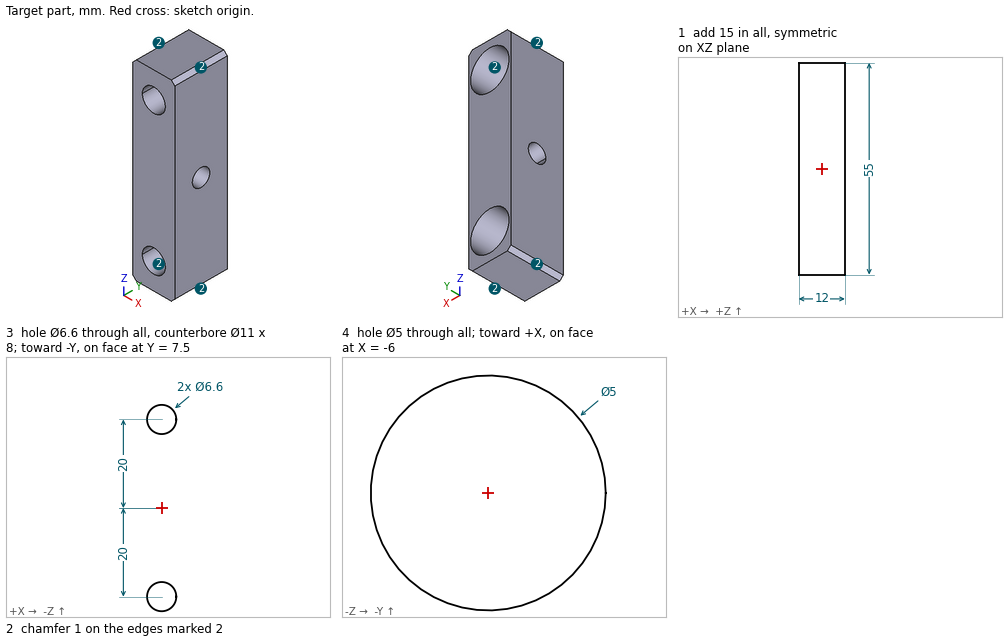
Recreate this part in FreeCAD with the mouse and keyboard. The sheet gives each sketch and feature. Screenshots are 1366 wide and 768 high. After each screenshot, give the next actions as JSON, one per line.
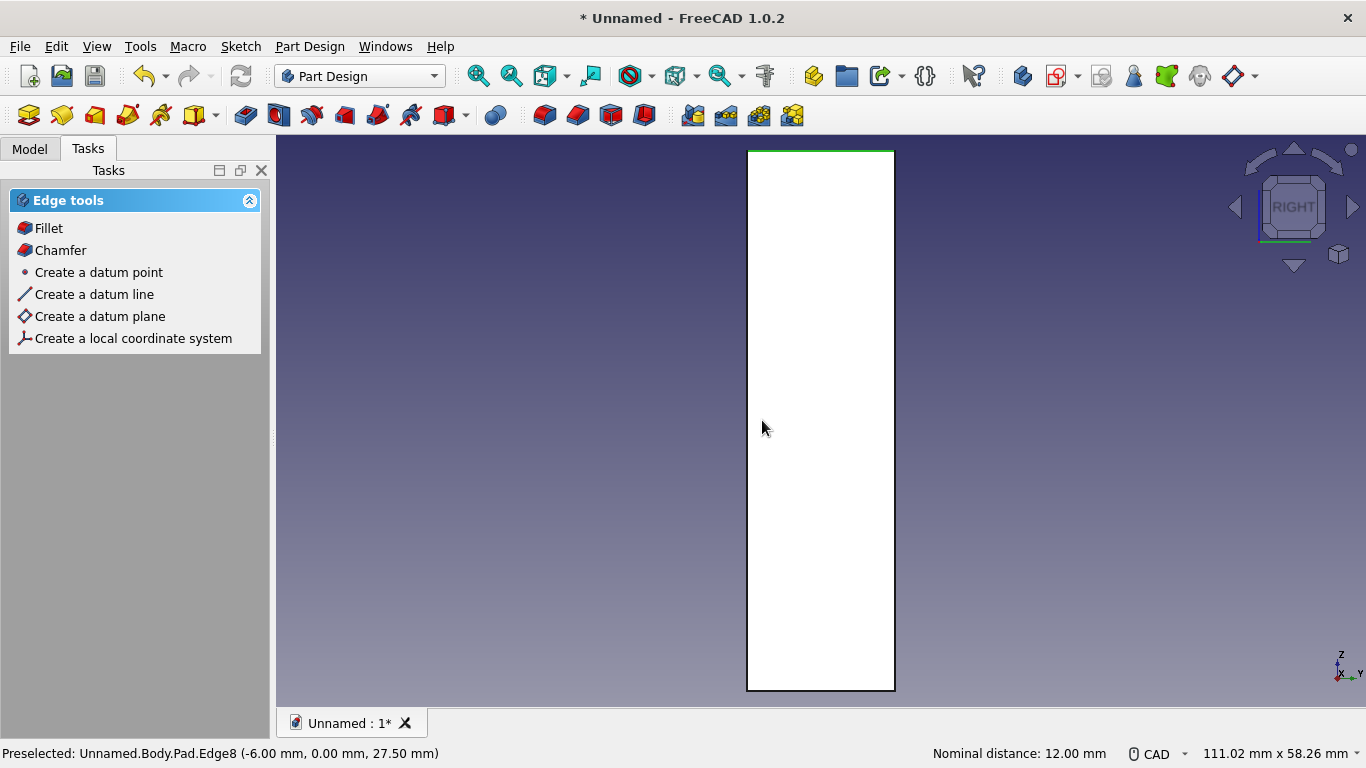
{"action": "key", "text": "5"}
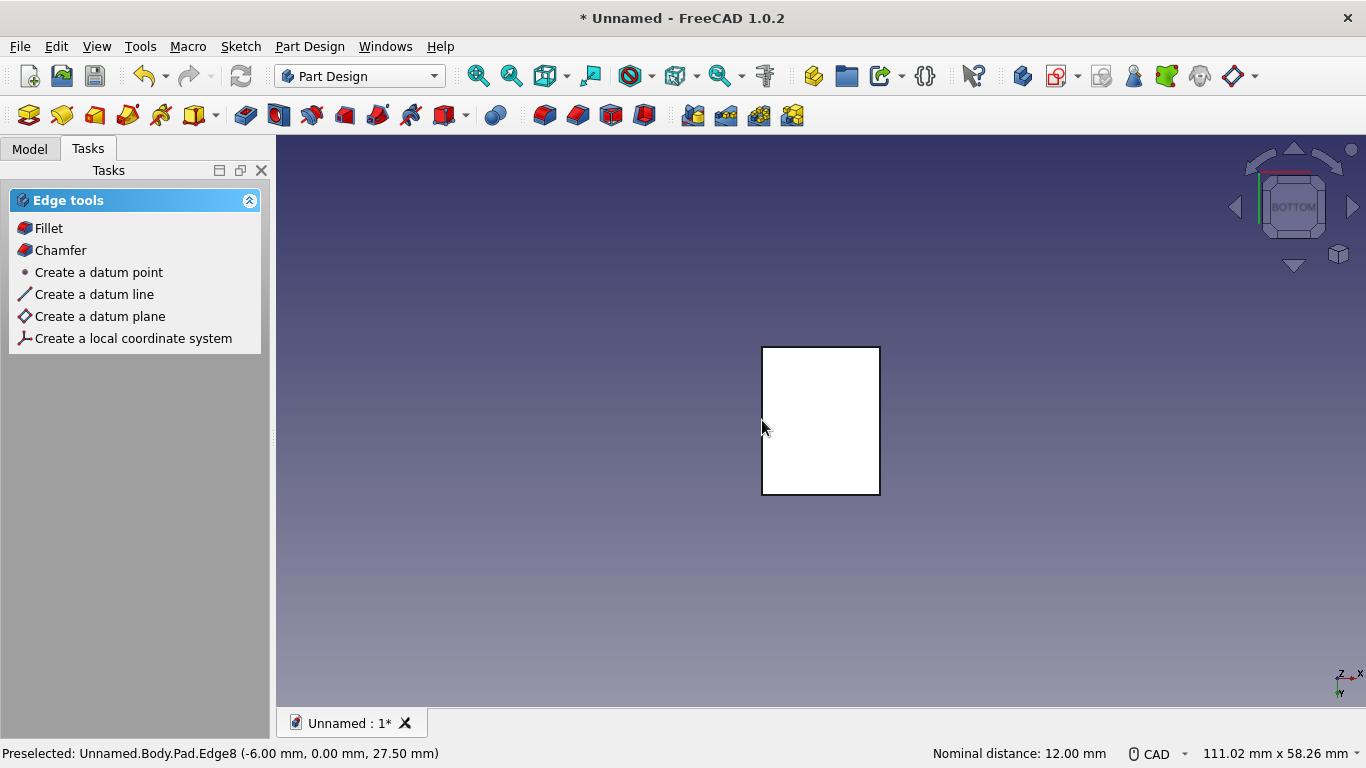
{"action": "left_click", "coordinate": [479, 76]}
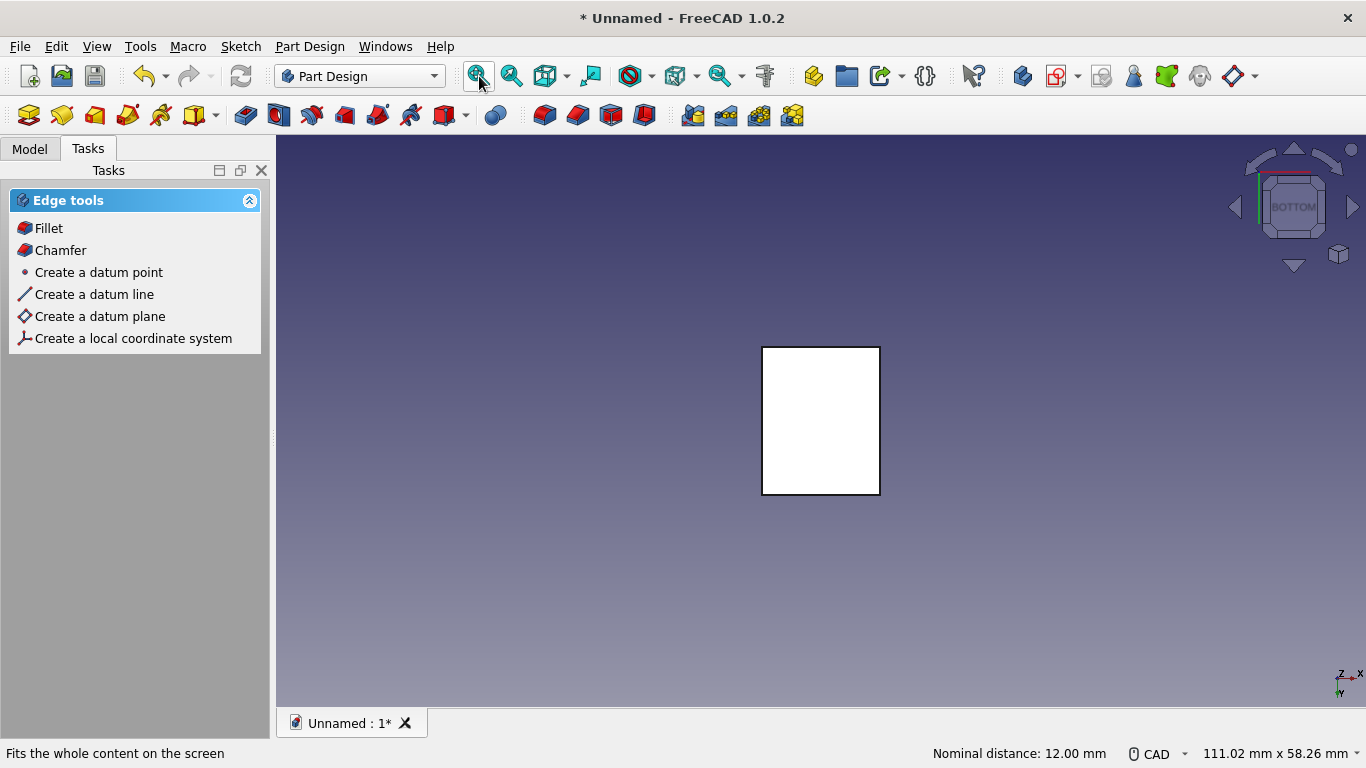
{"action": "left_click", "coordinate": [762, 420], "text": "ctrl"}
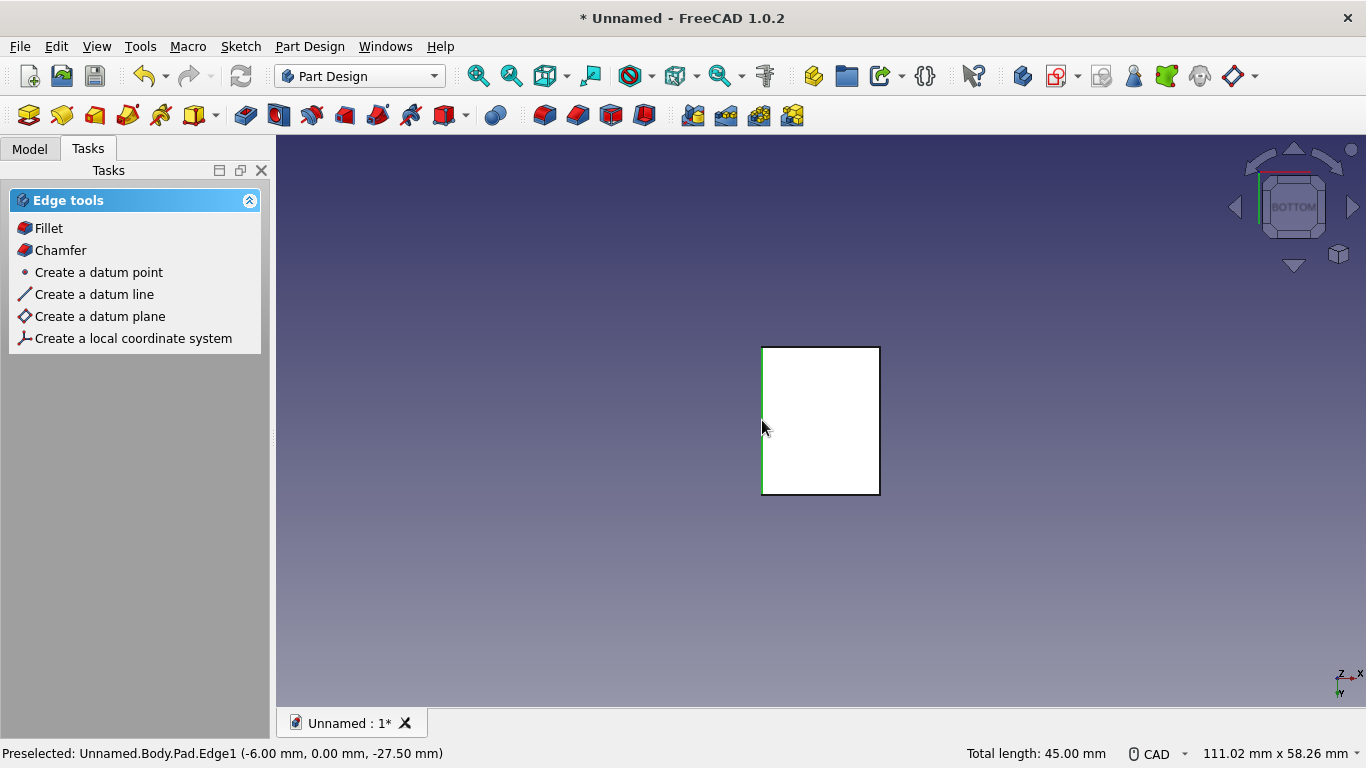
{"action": "left_click", "coordinate": [880, 420], "text": "ctrl"}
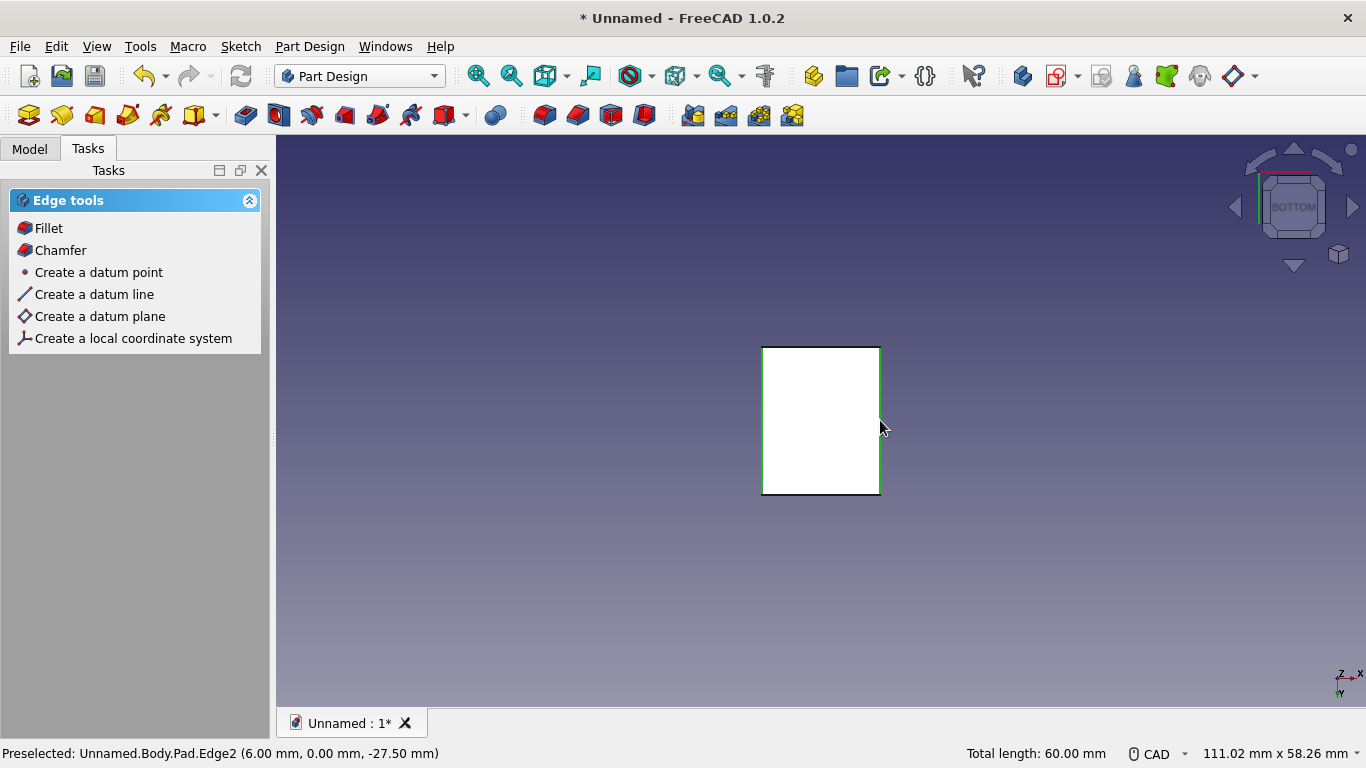
{"action": "left_click", "coordinate": [578, 116]}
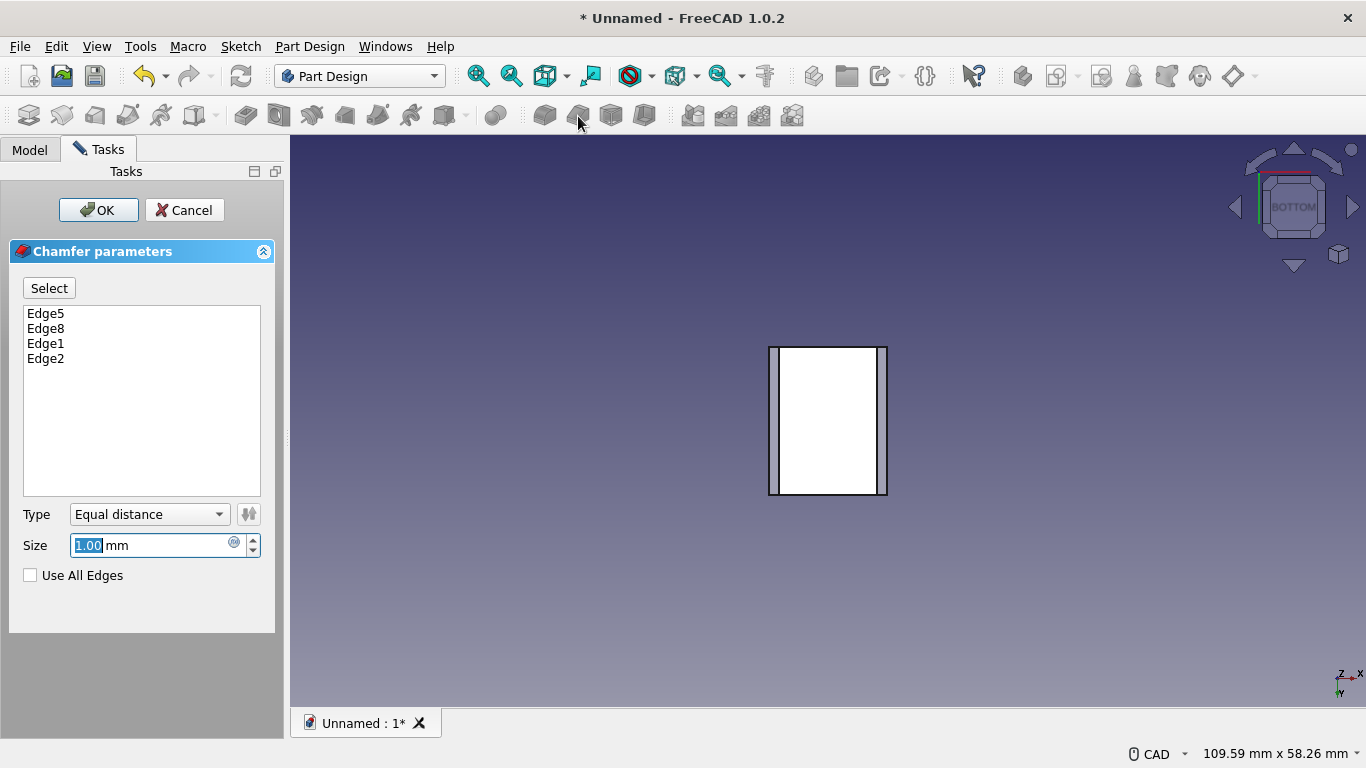
{"action": "type", "text": "1"}
{"action": "key", "text": "Tab"}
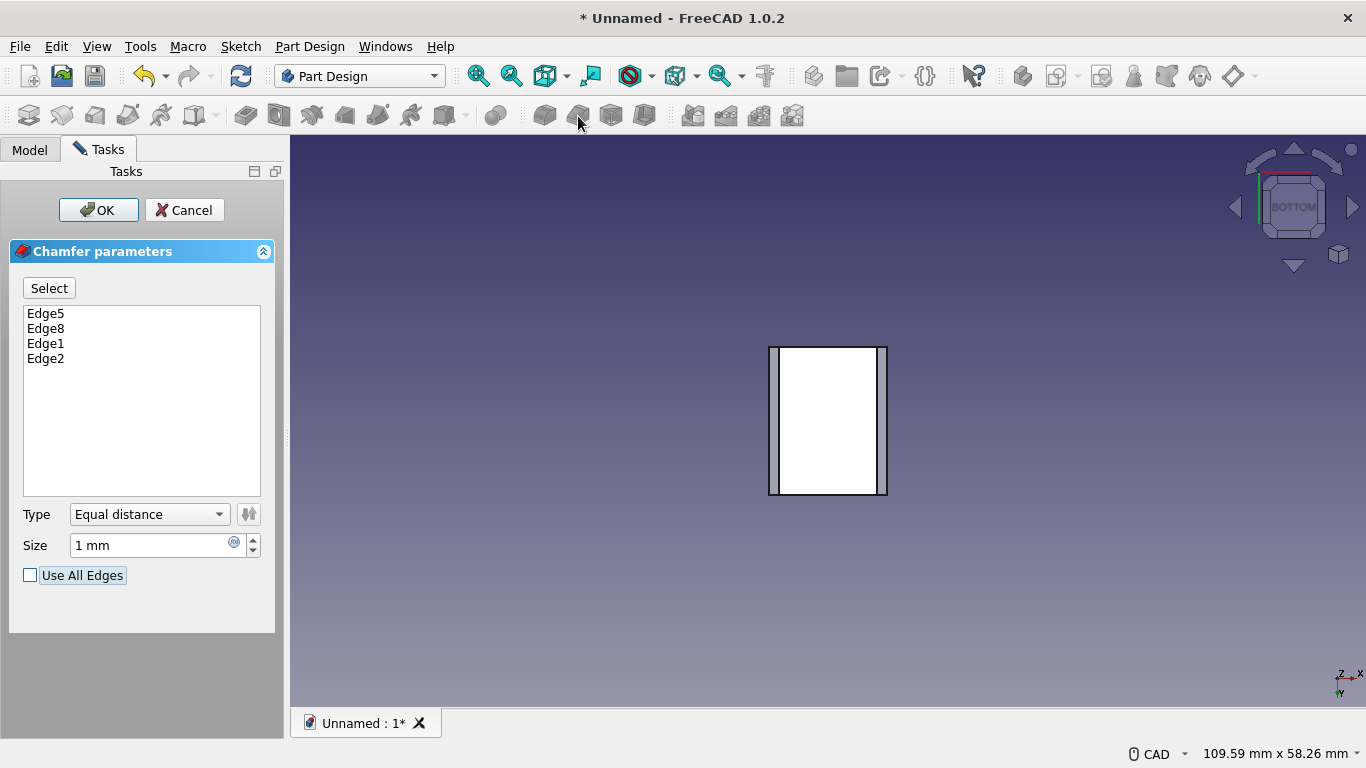
{"action": "left_click", "coordinate": [99, 210]}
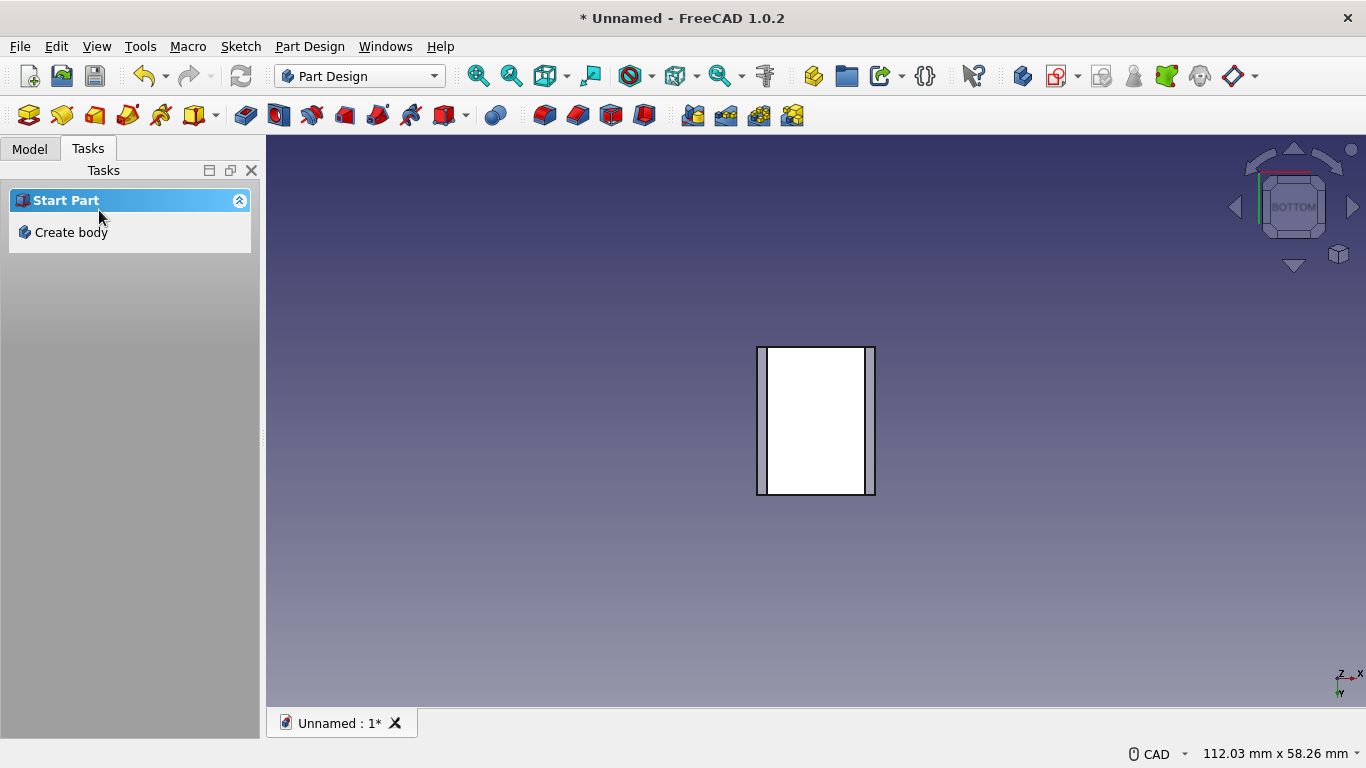
{"action": "left_click", "coordinate": [479, 76]}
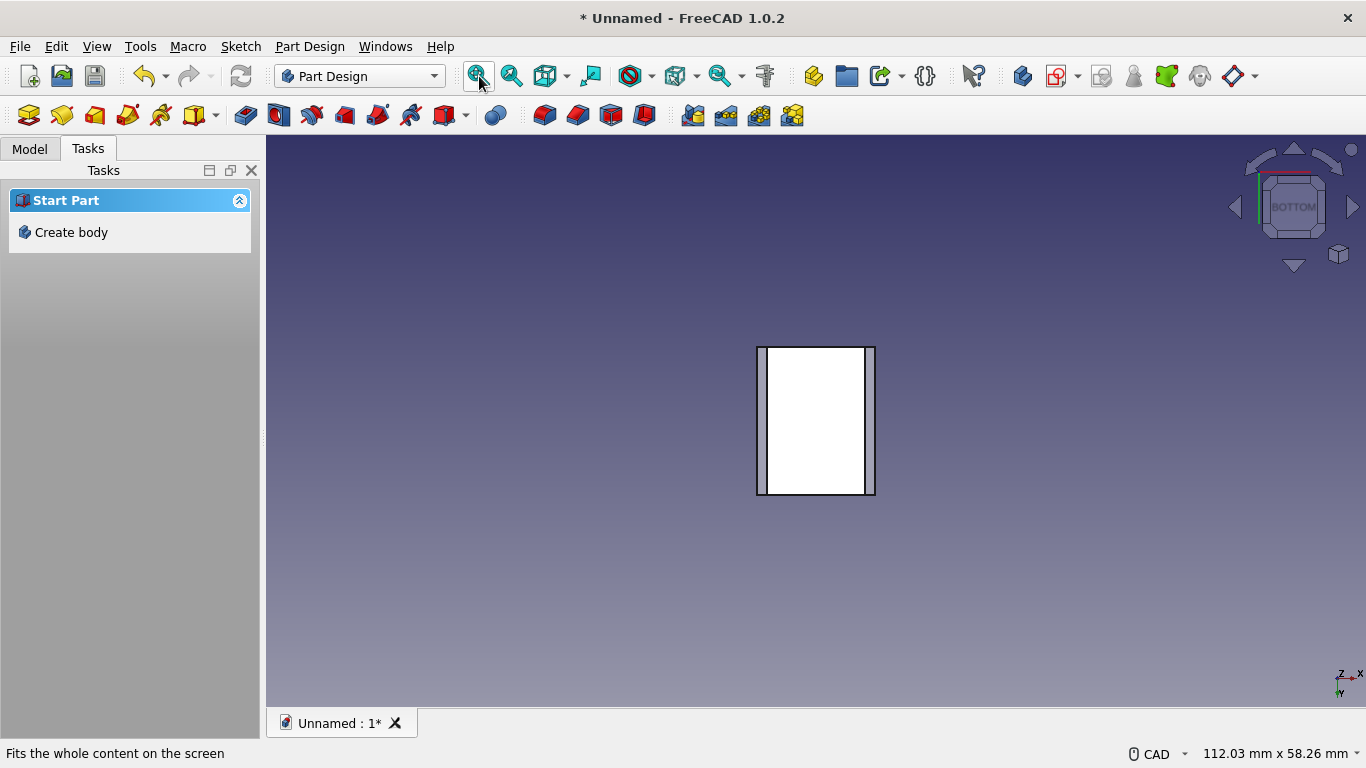
{"action": "key", "text": "4"}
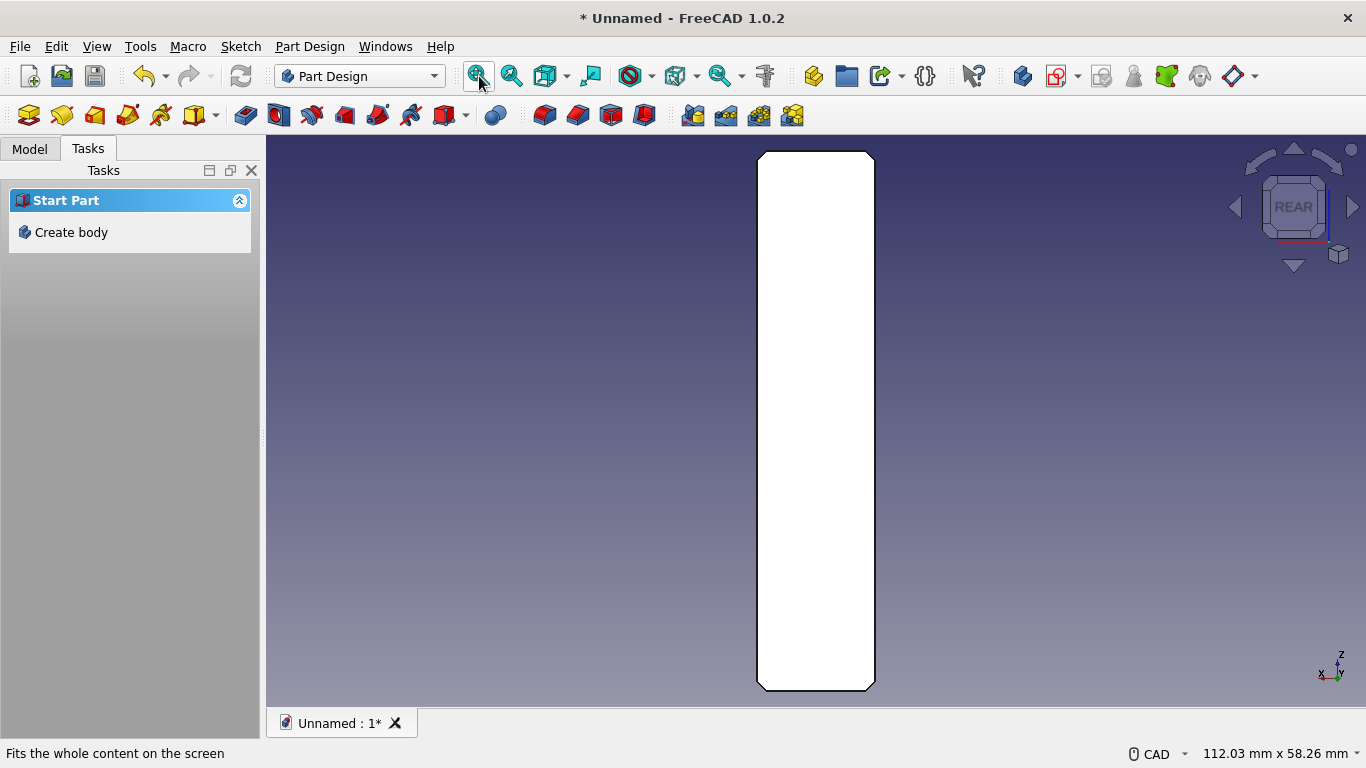
{"action": "left_click", "coordinate": [816, 266]}